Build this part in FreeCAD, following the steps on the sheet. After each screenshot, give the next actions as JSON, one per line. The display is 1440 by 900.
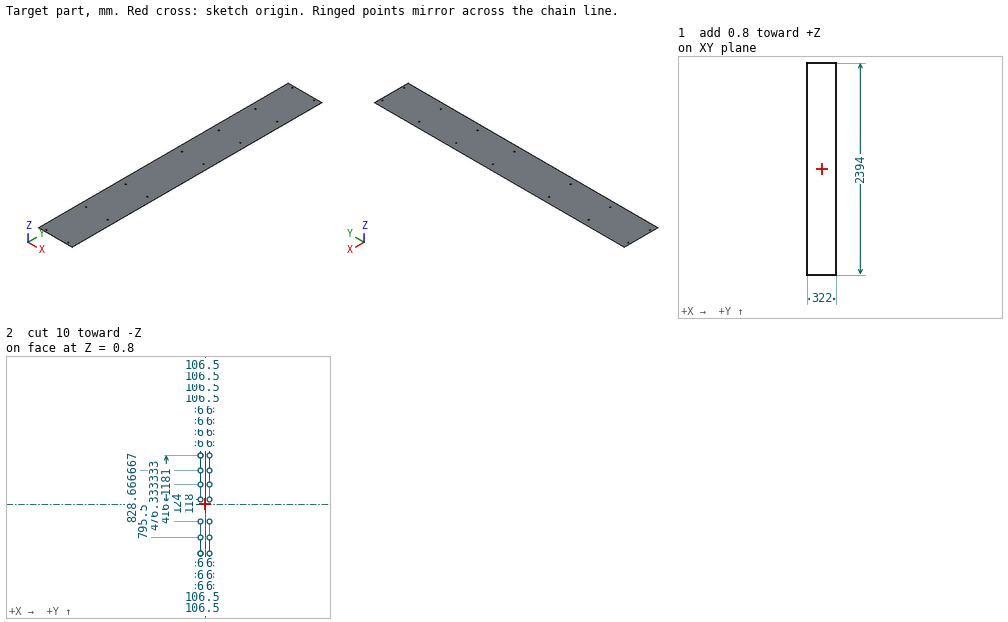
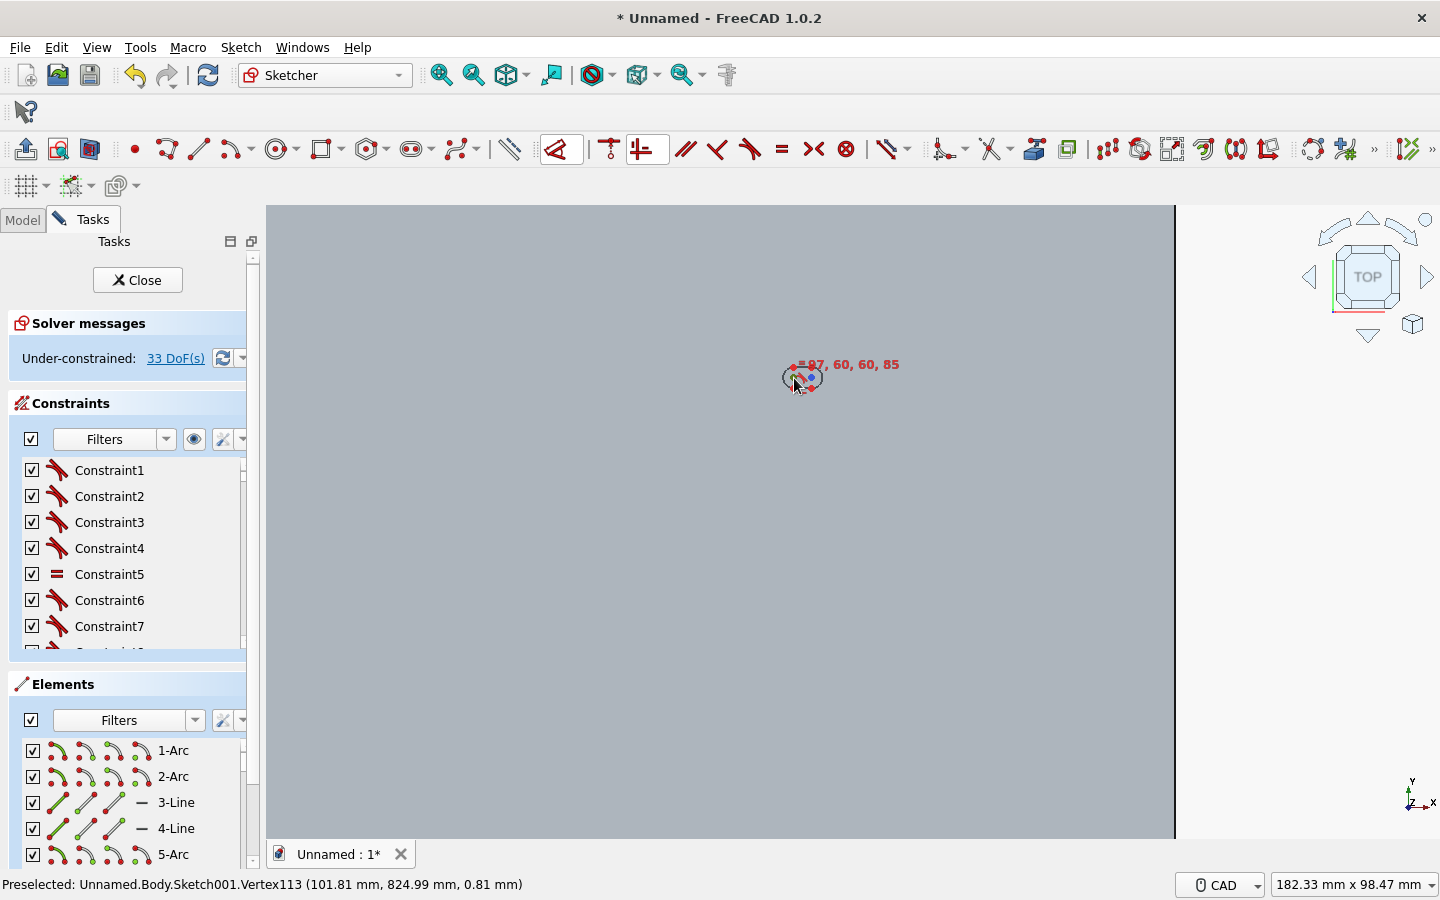
{"action": "scroll", "coordinate": [807, 344], "scroll_direction": "down", "scroll_amount": 17}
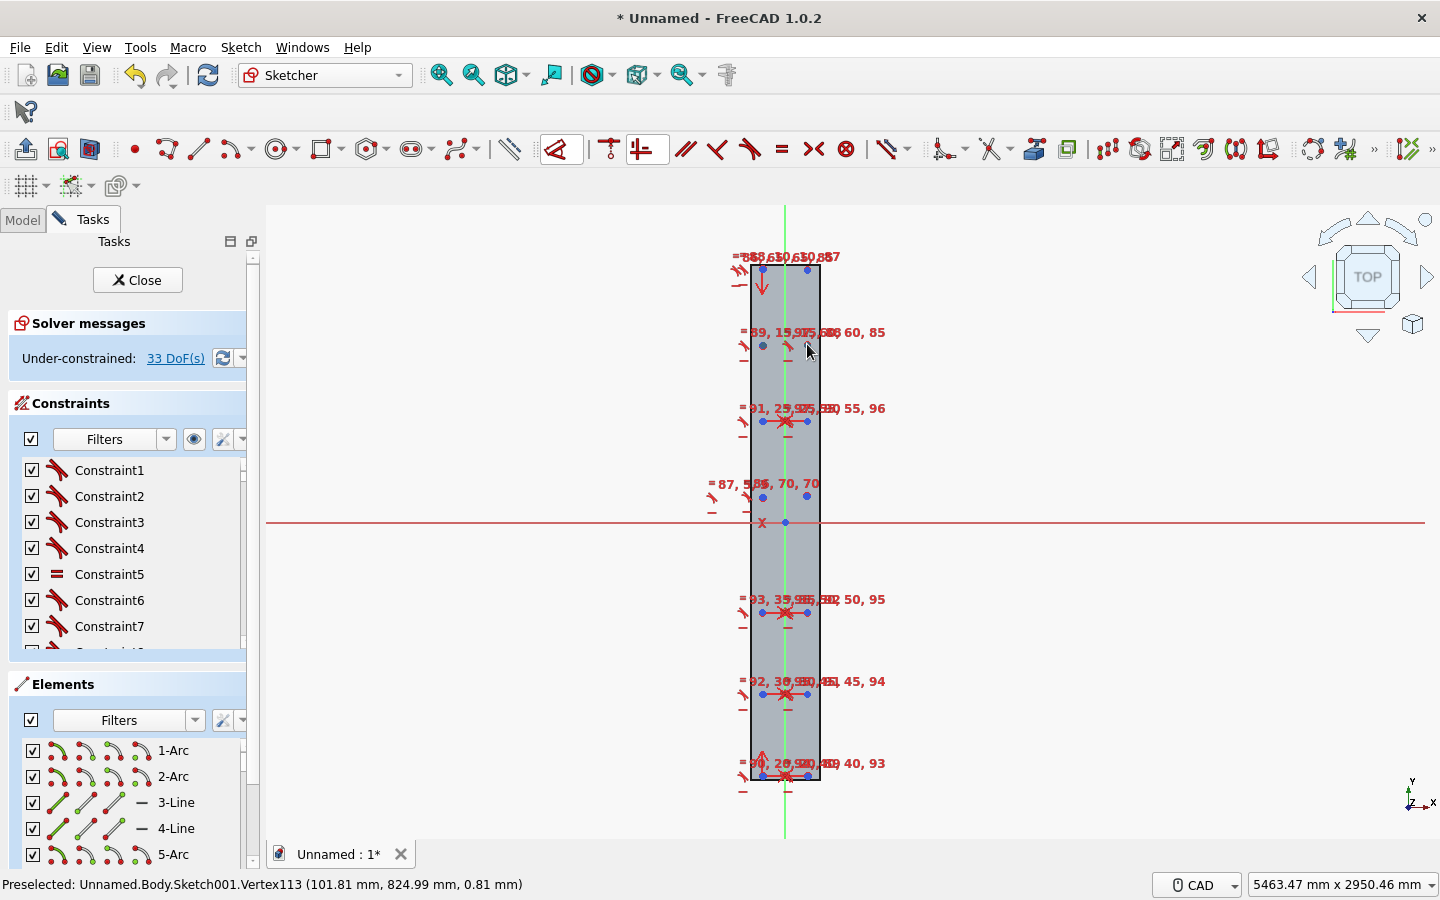
{"action": "left_click", "coordinate": [785, 728]}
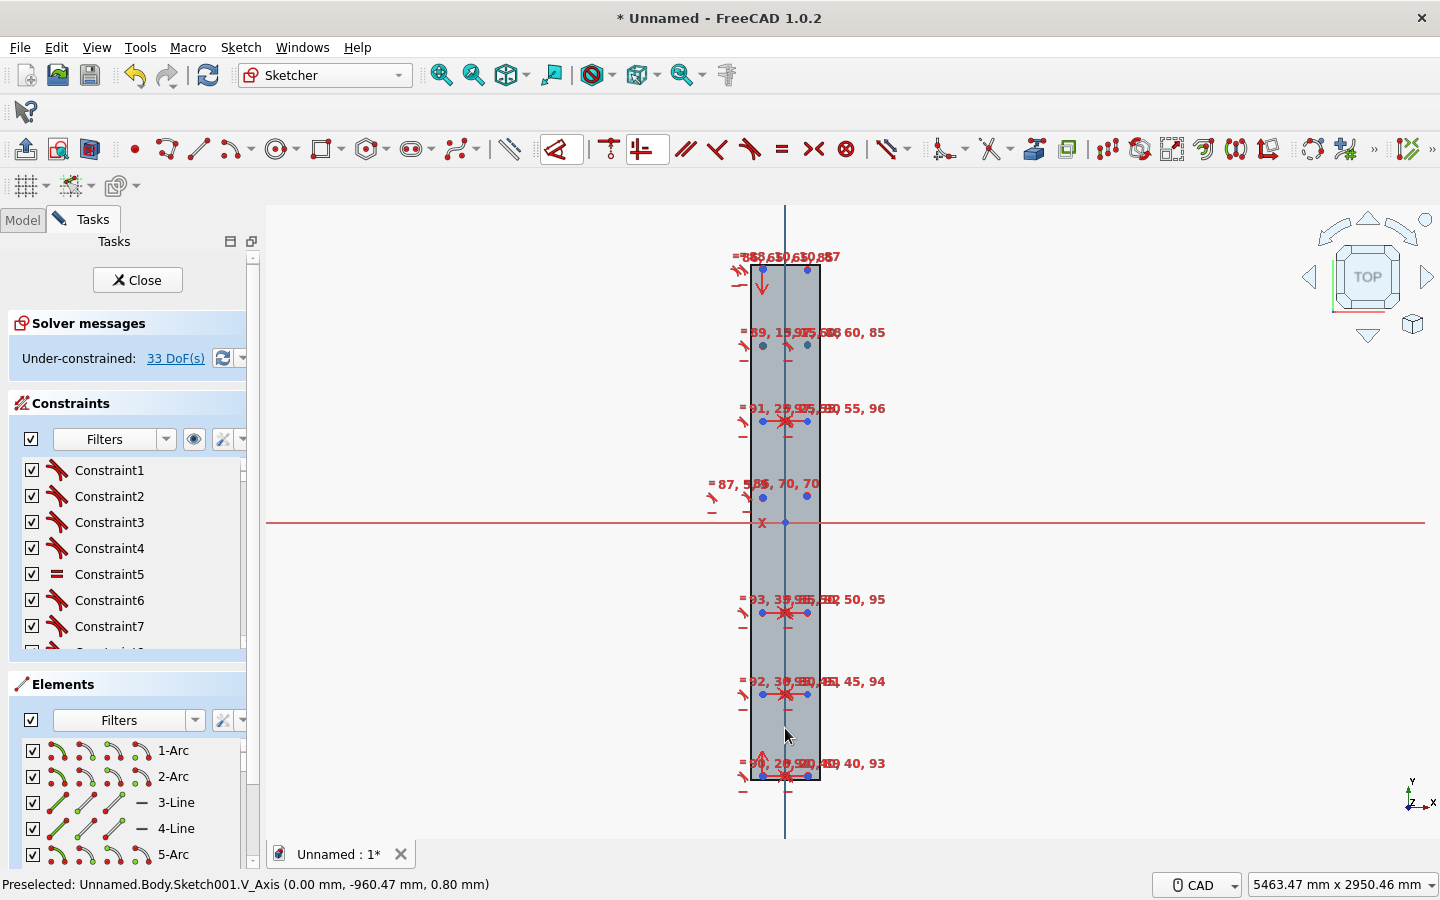
{"action": "key", "text": "s"}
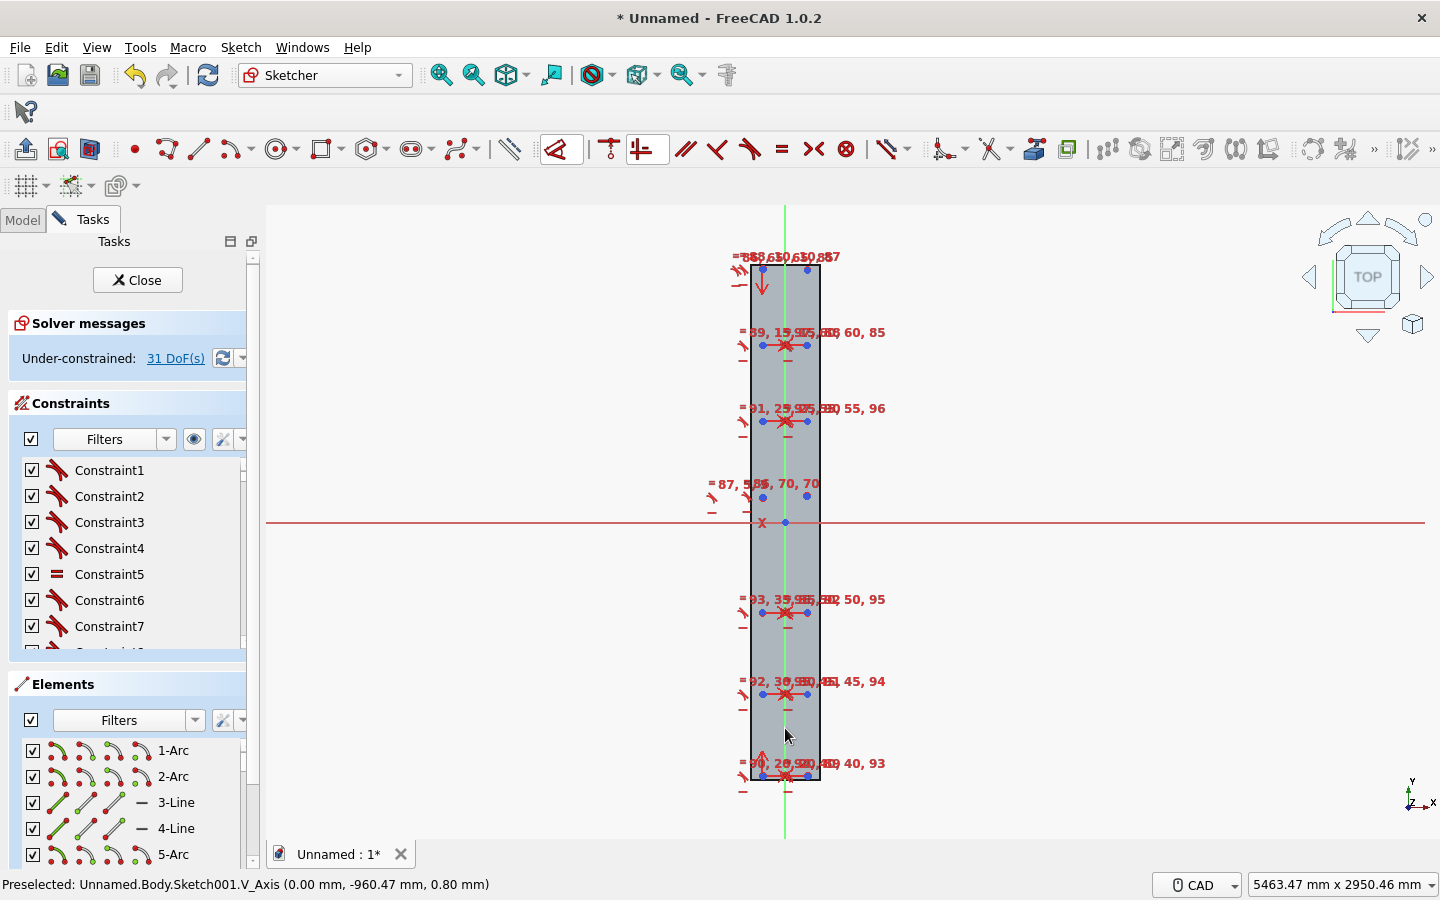
{"action": "scroll", "coordinate": [763, 269], "scroll_direction": "up", "scroll_amount": 13}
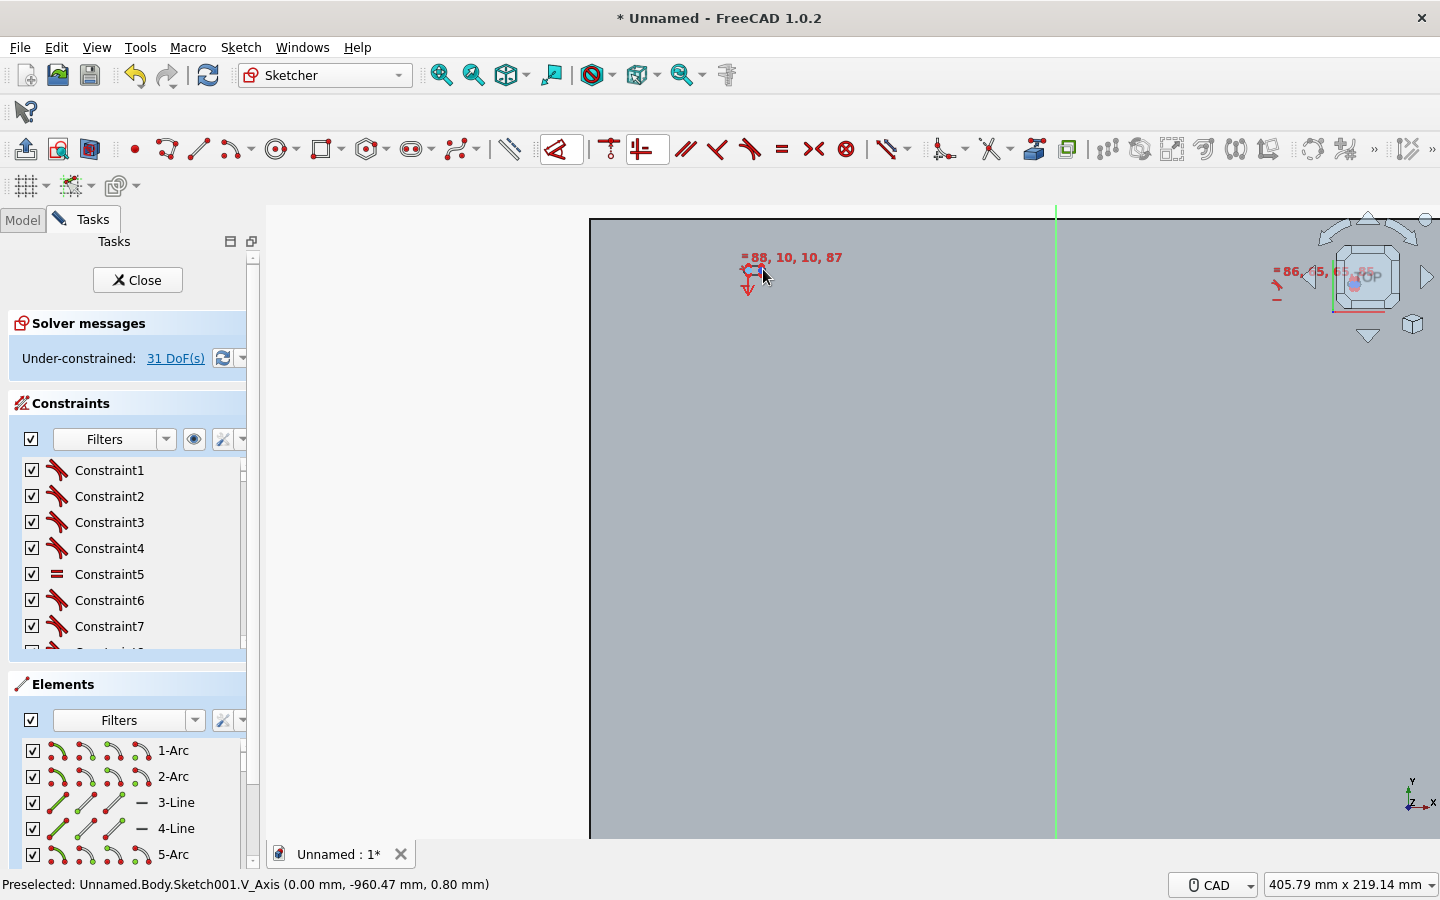
{"action": "left_click", "coordinate": [761, 271]}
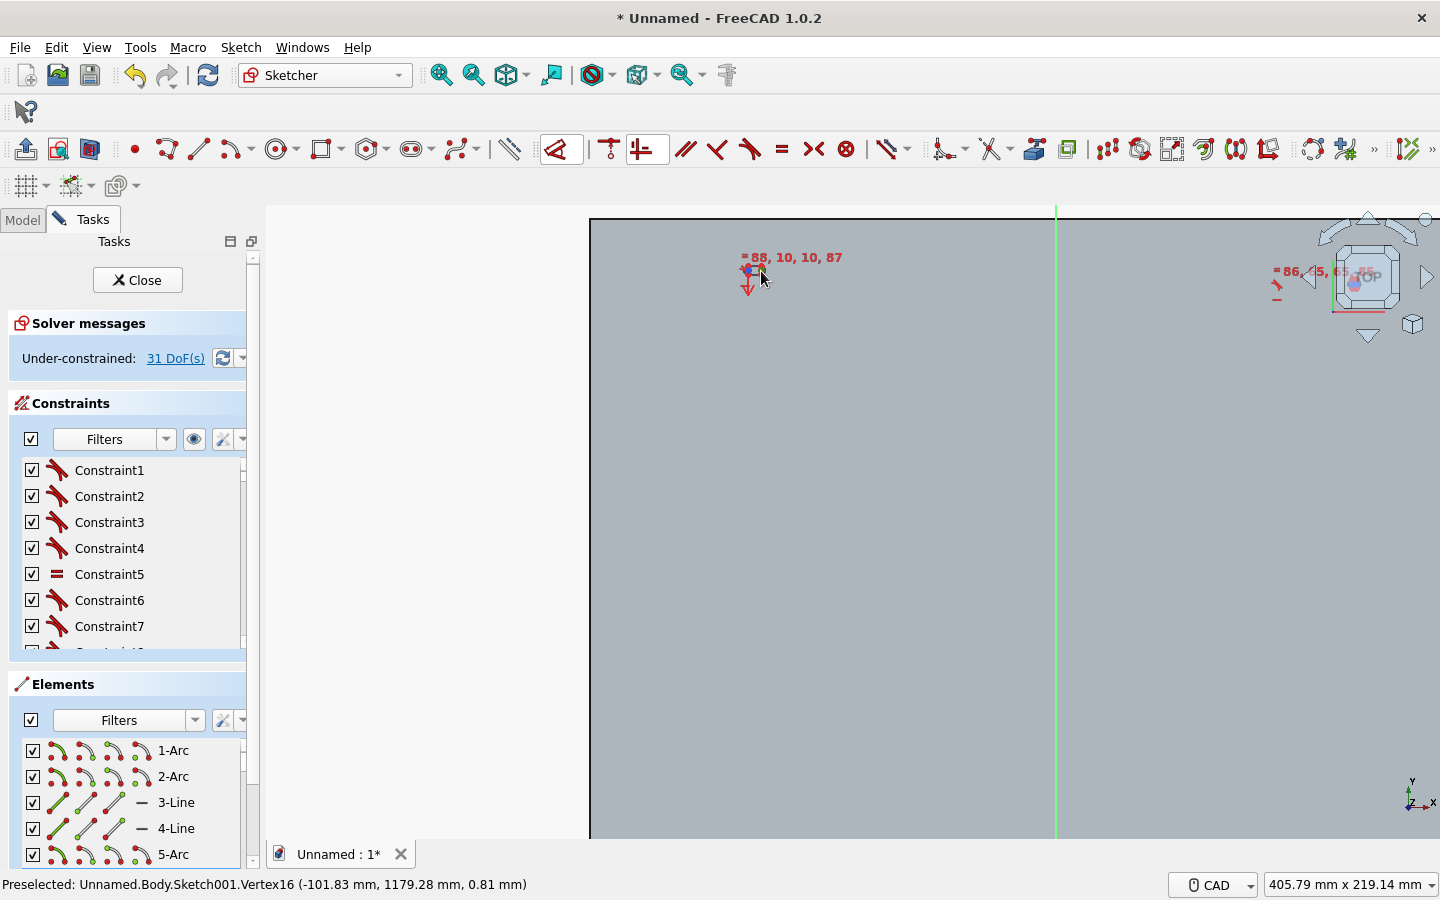
{"action": "scroll", "coordinate": [767, 317], "scroll_direction": "down", "scroll_amount": 14}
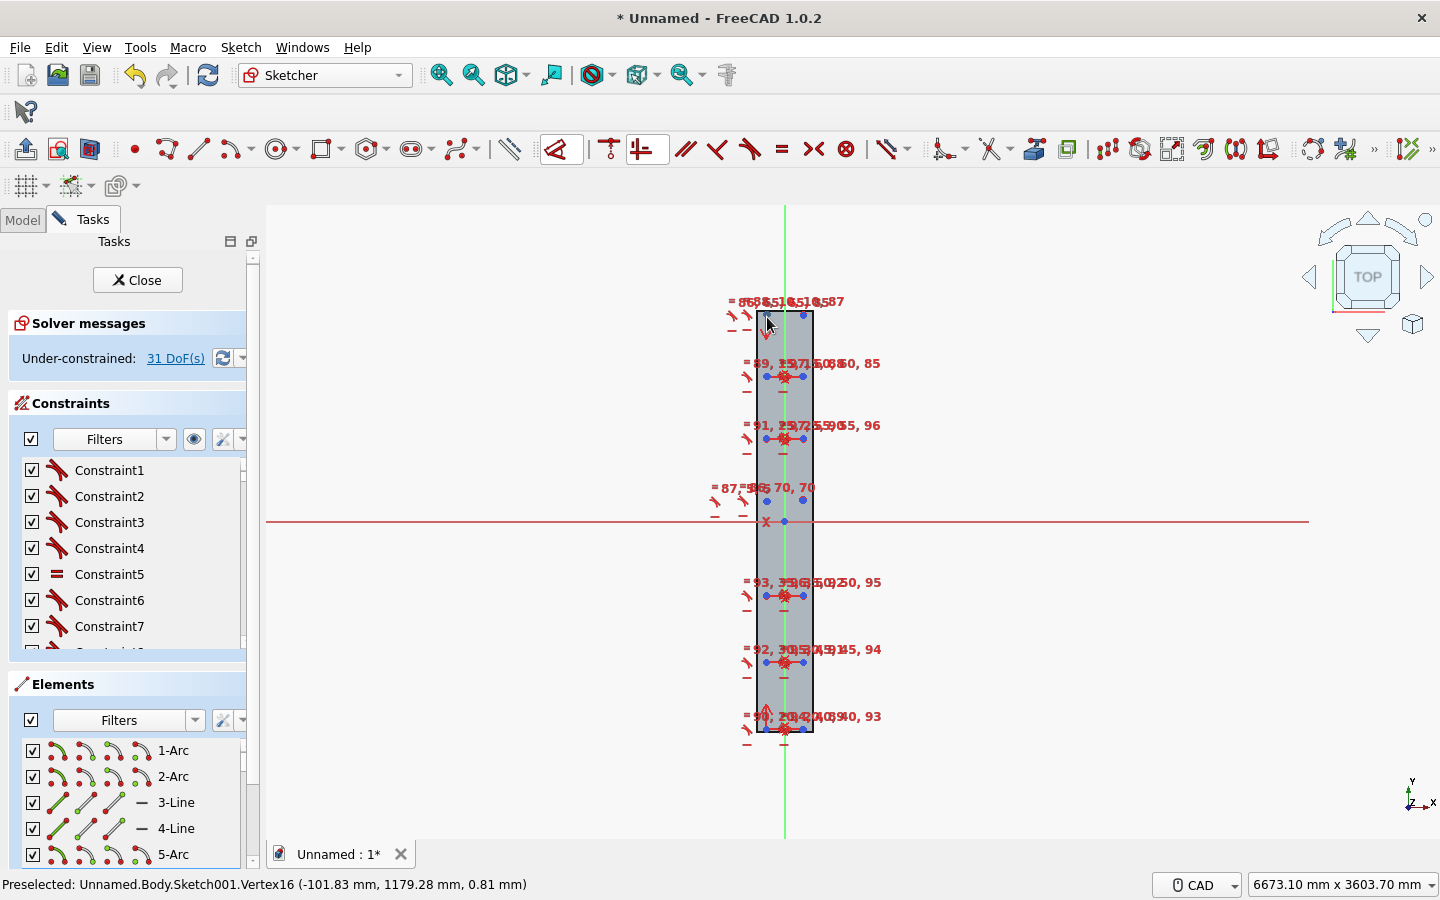
{"action": "scroll", "coordinate": [803, 315], "scroll_direction": "up", "scroll_amount": 14}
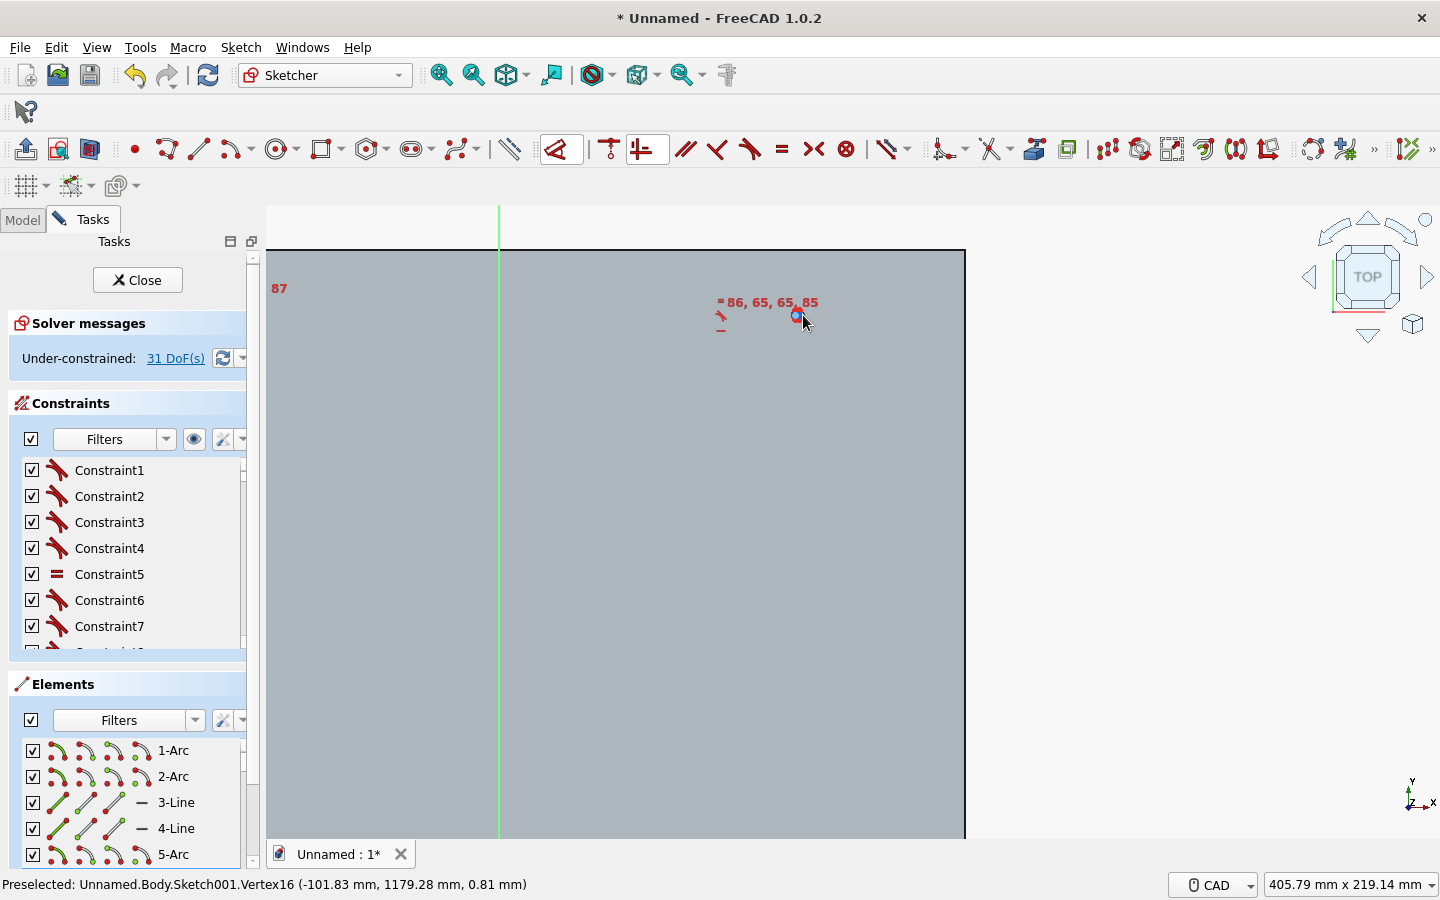
{"action": "left_click", "coordinate": [796, 315]}